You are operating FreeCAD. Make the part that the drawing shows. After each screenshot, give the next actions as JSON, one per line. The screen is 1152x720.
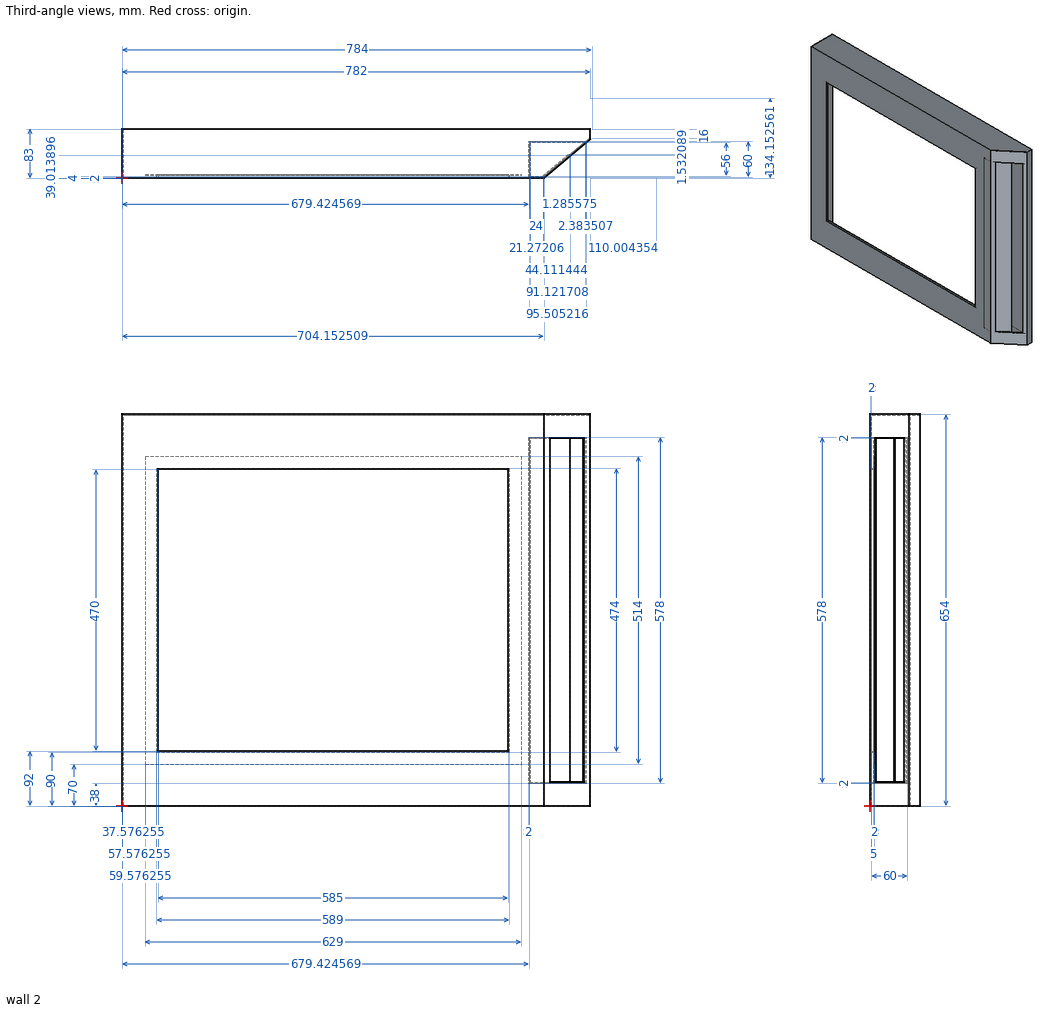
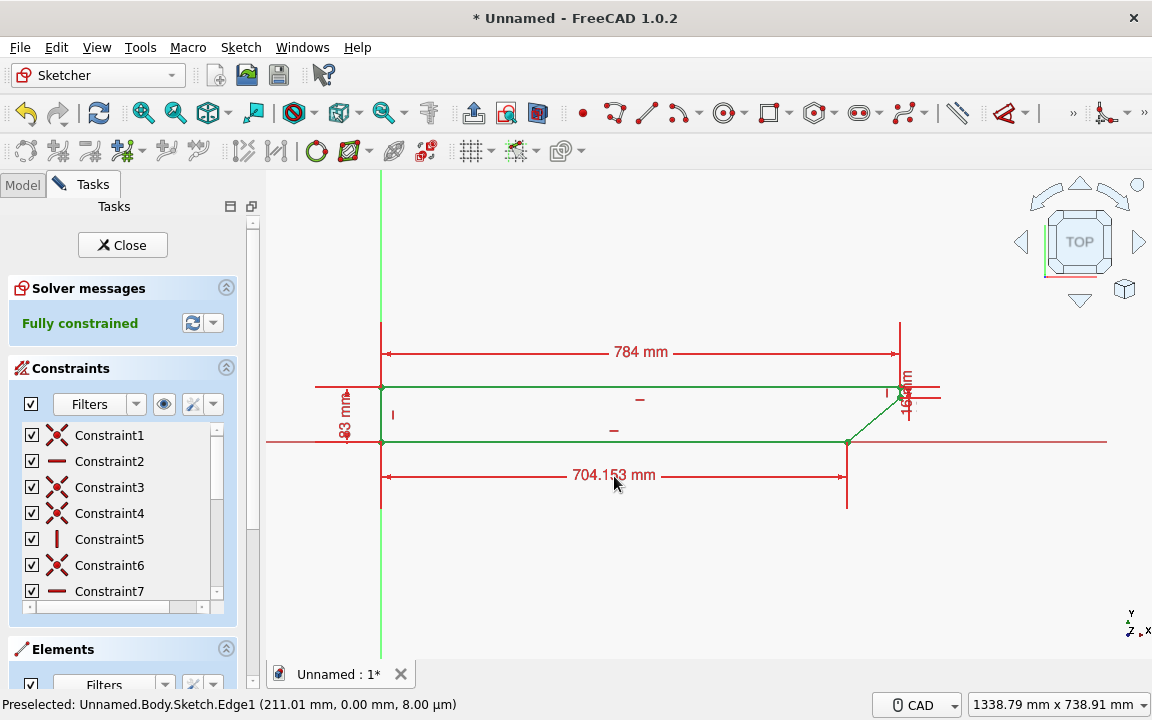
{"action": "left_click", "coordinate": [123, 245]}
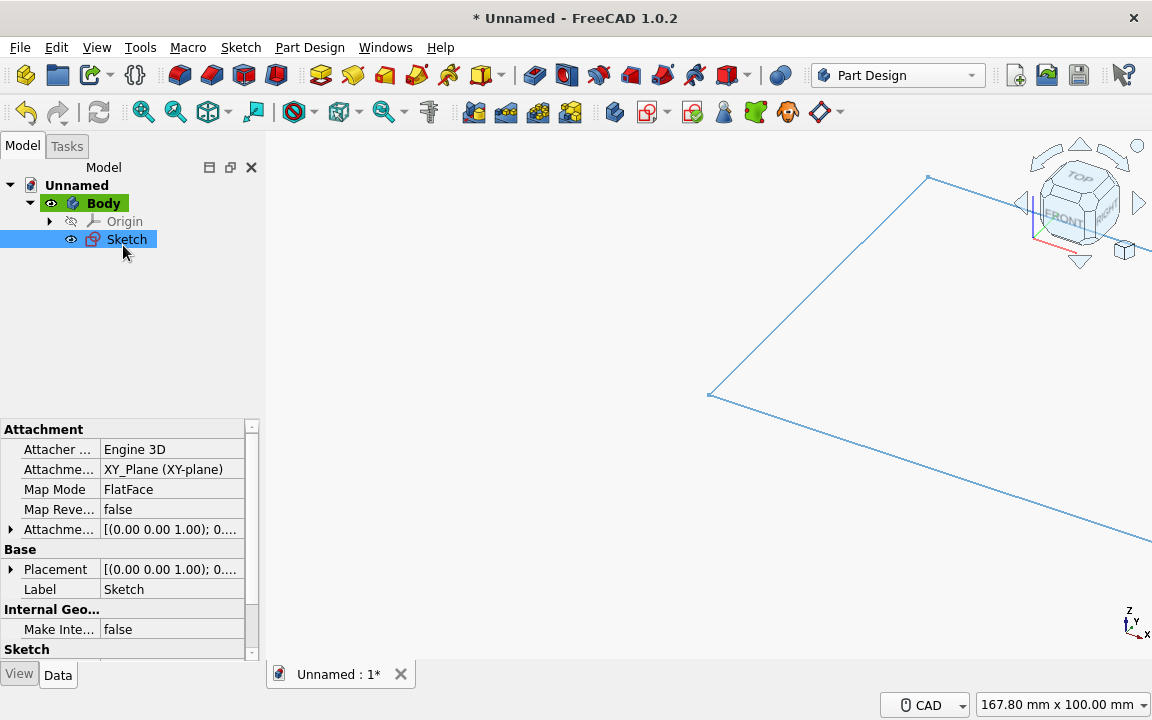
{"action": "left_click", "coordinate": [322, 76]}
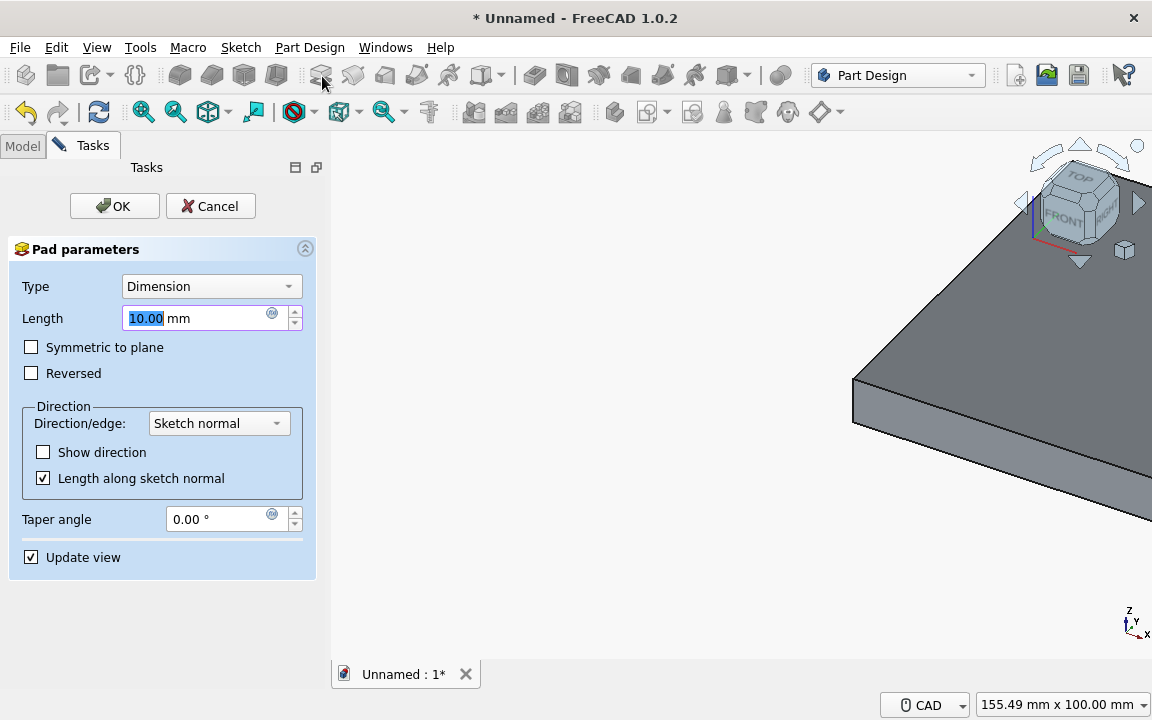
{"action": "type", "text": "654"}
{"action": "key", "text": "Tab"}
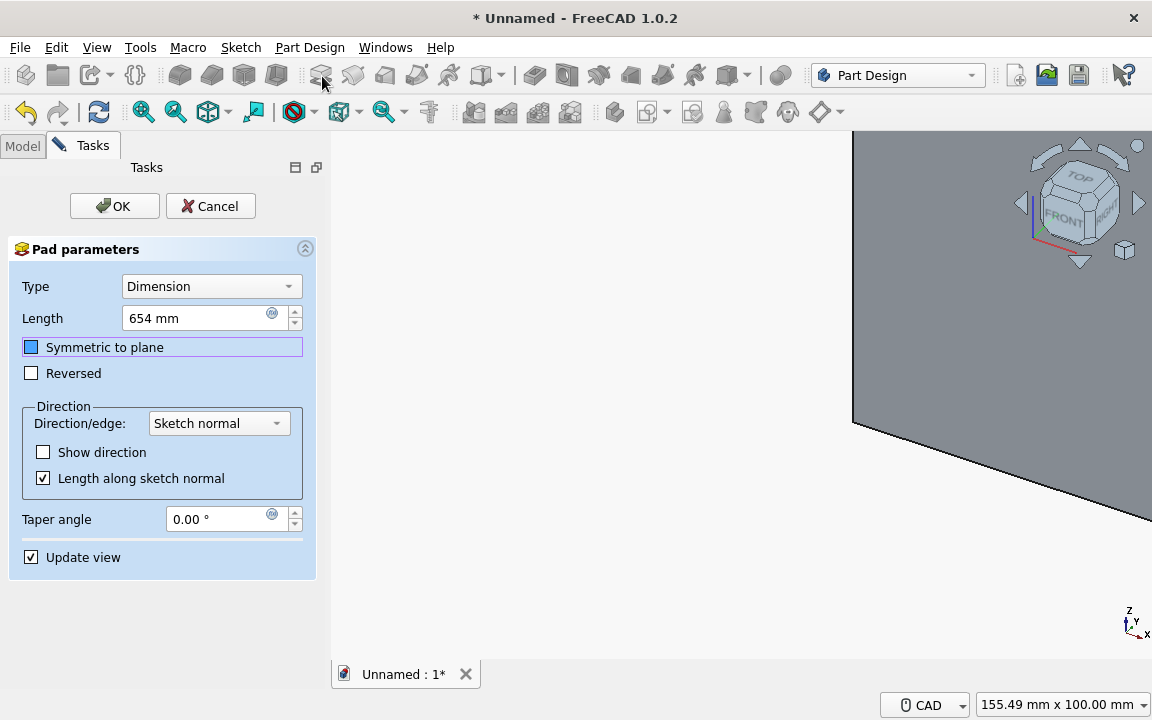
{"action": "left_click", "coordinate": [115, 206]}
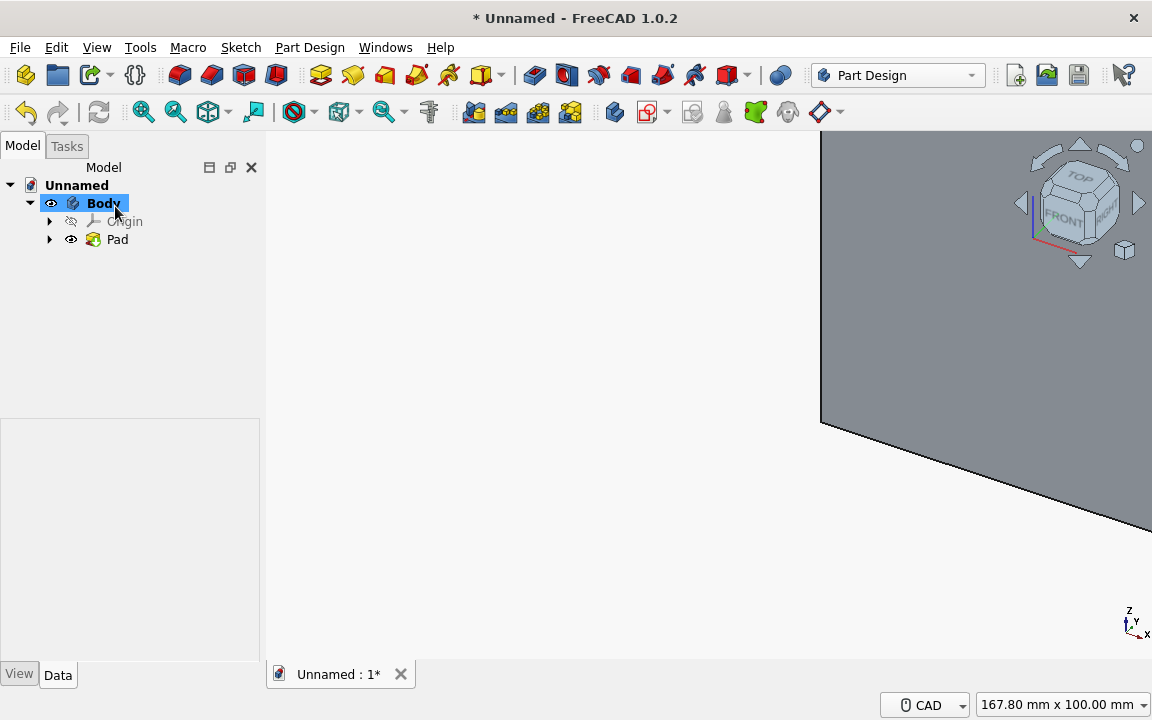
{"action": "key", "text": "v f"}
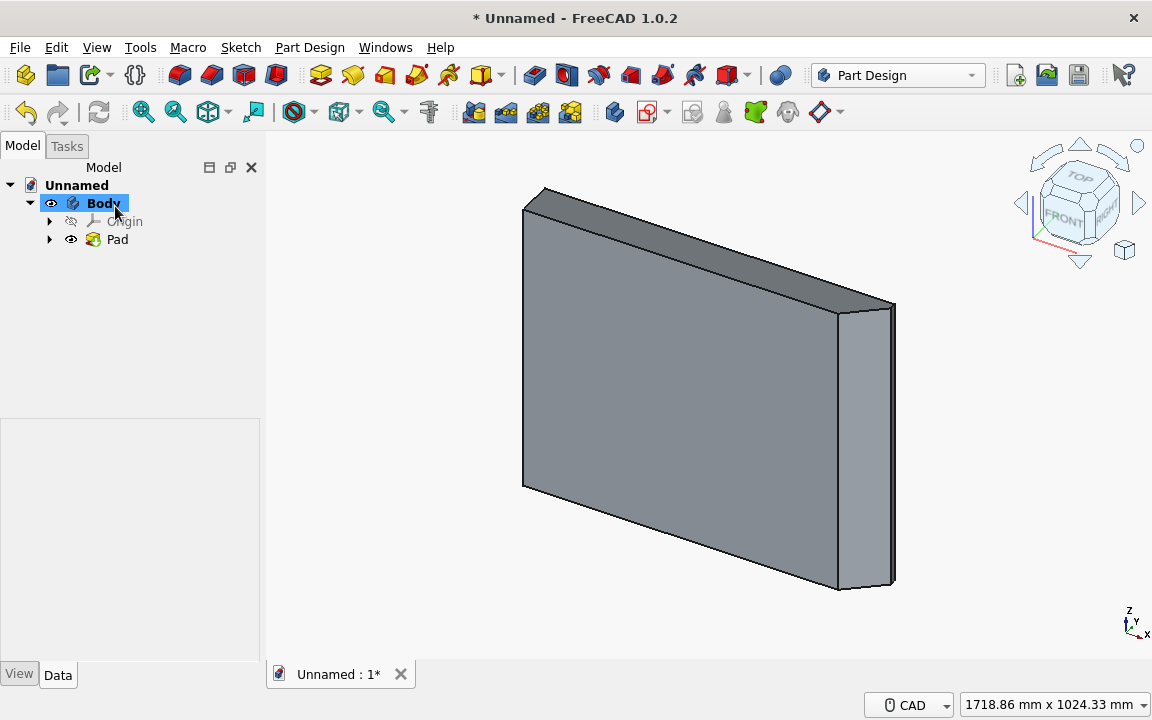
{"action": "left_click", "coordinate": [809, 289]}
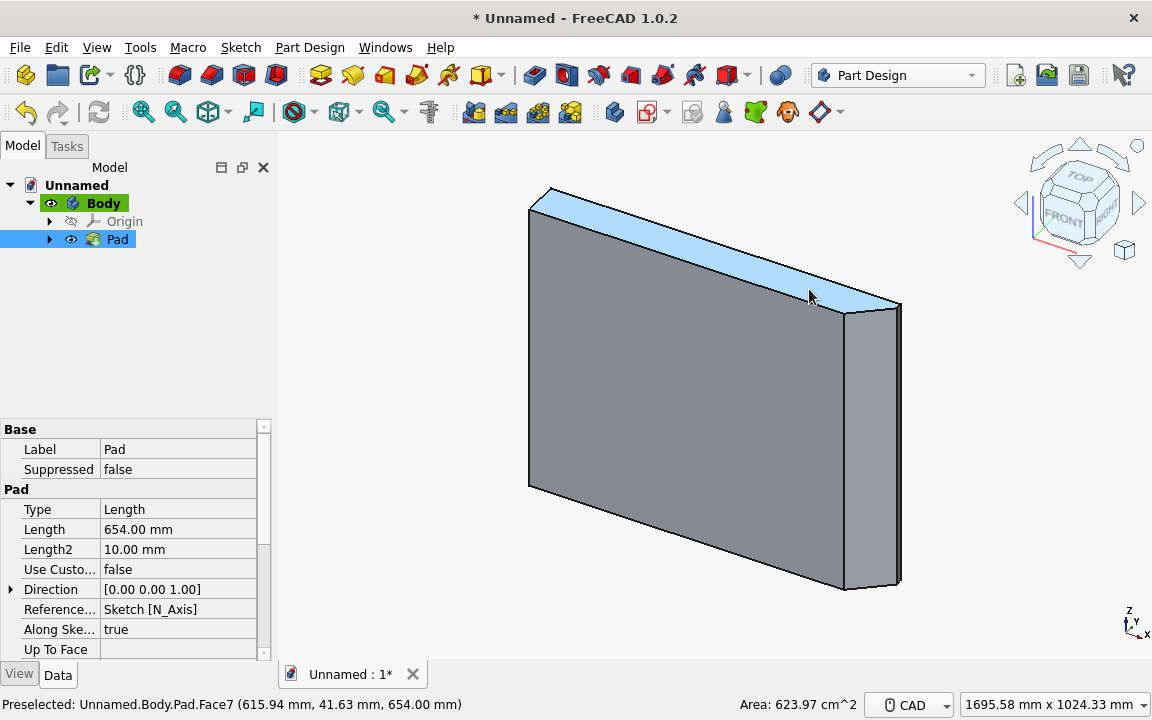
{"action": "left_click", "coordinate": [648, 112]}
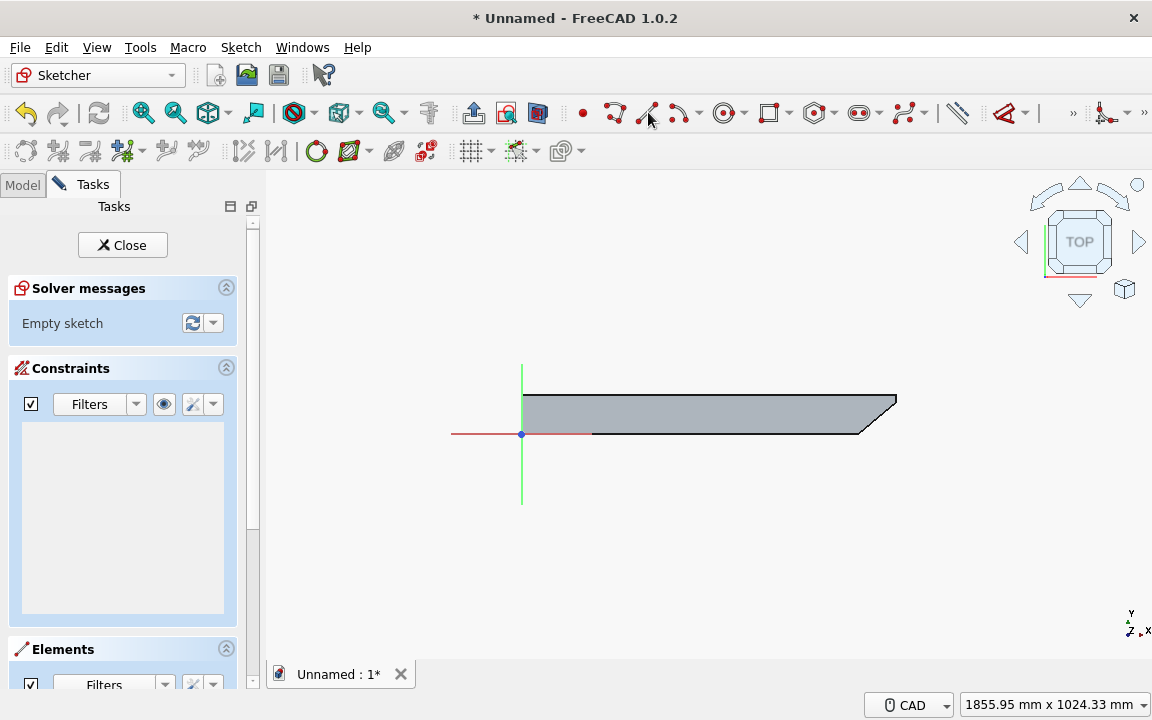
{"action": "scroll", "coordinate": [987, 399], "scroll_direction": "up", "scroll_amount": 8}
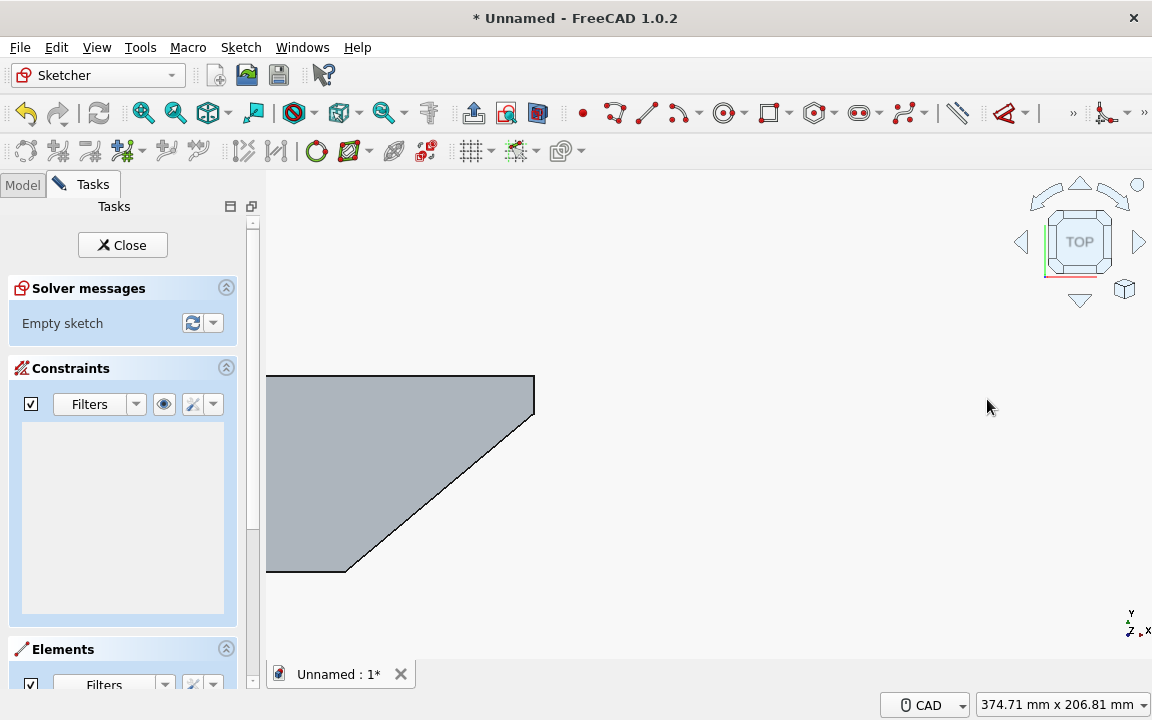
{"action": "key", "text": "g r"}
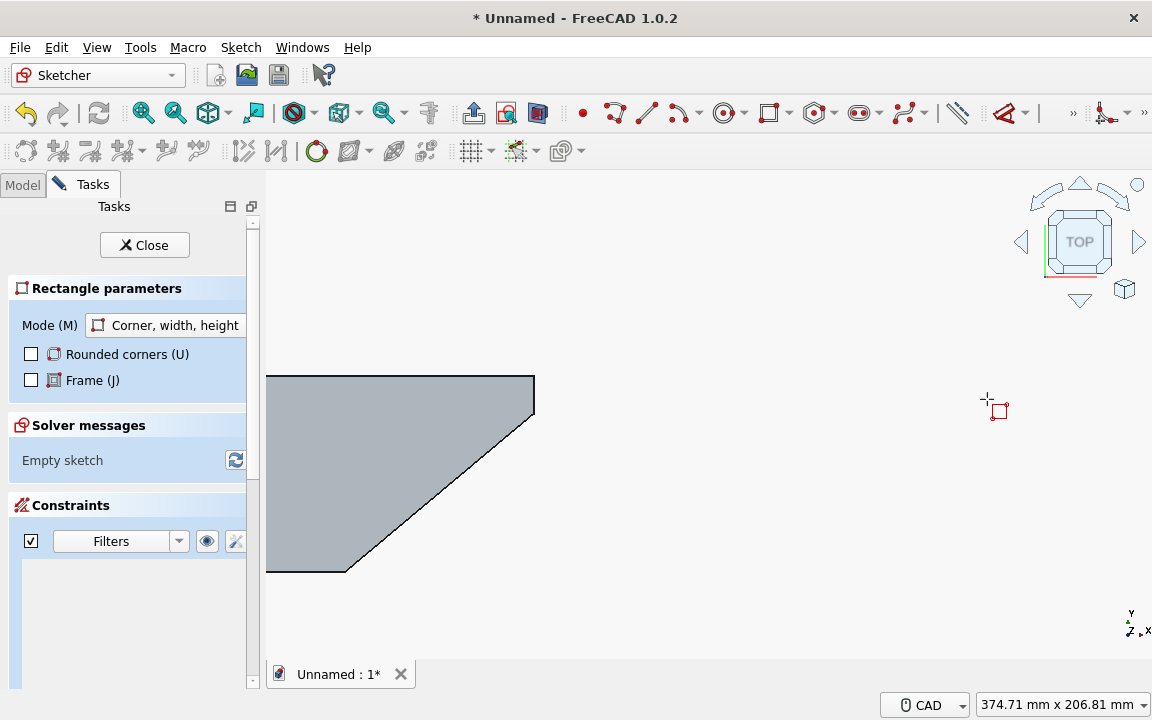
{"action": "left_click", "coordinate": [529, 255]}
{"action": "left_click", "coordinate": [789, 572]}
{"action": "key", "text": "Escape"}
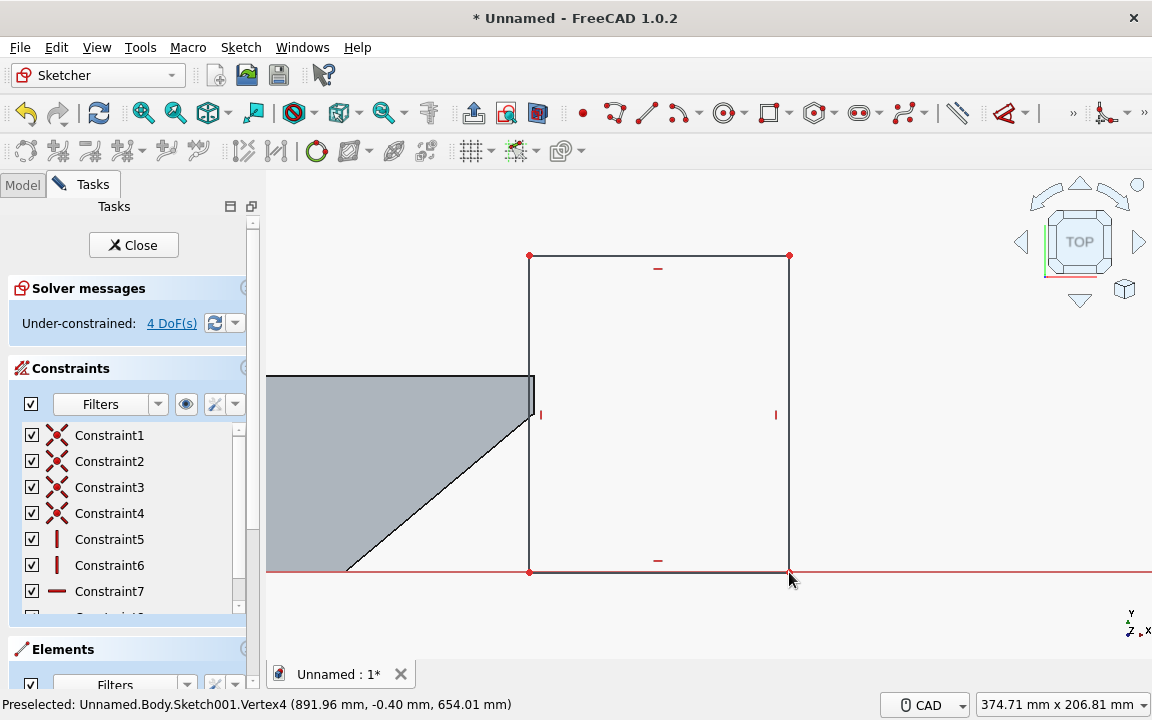
{"action": "left_click", "coordinate": [529, 573]}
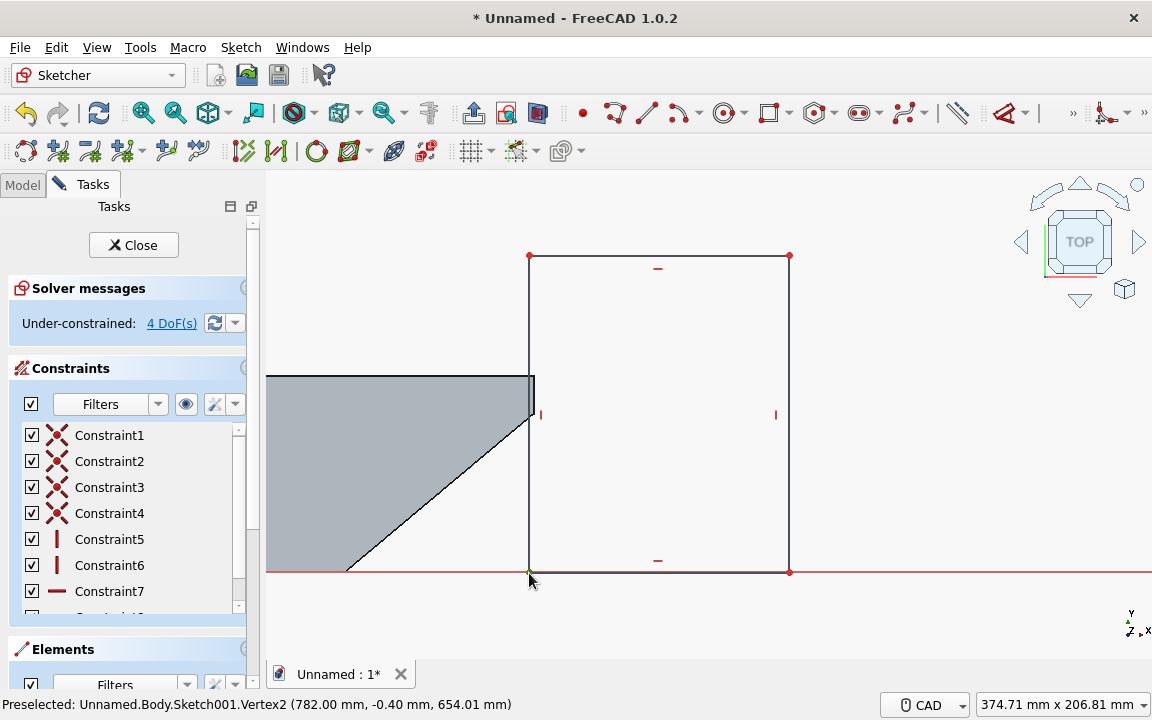
{"action": "left_click", "coordinate": [344, 572]}